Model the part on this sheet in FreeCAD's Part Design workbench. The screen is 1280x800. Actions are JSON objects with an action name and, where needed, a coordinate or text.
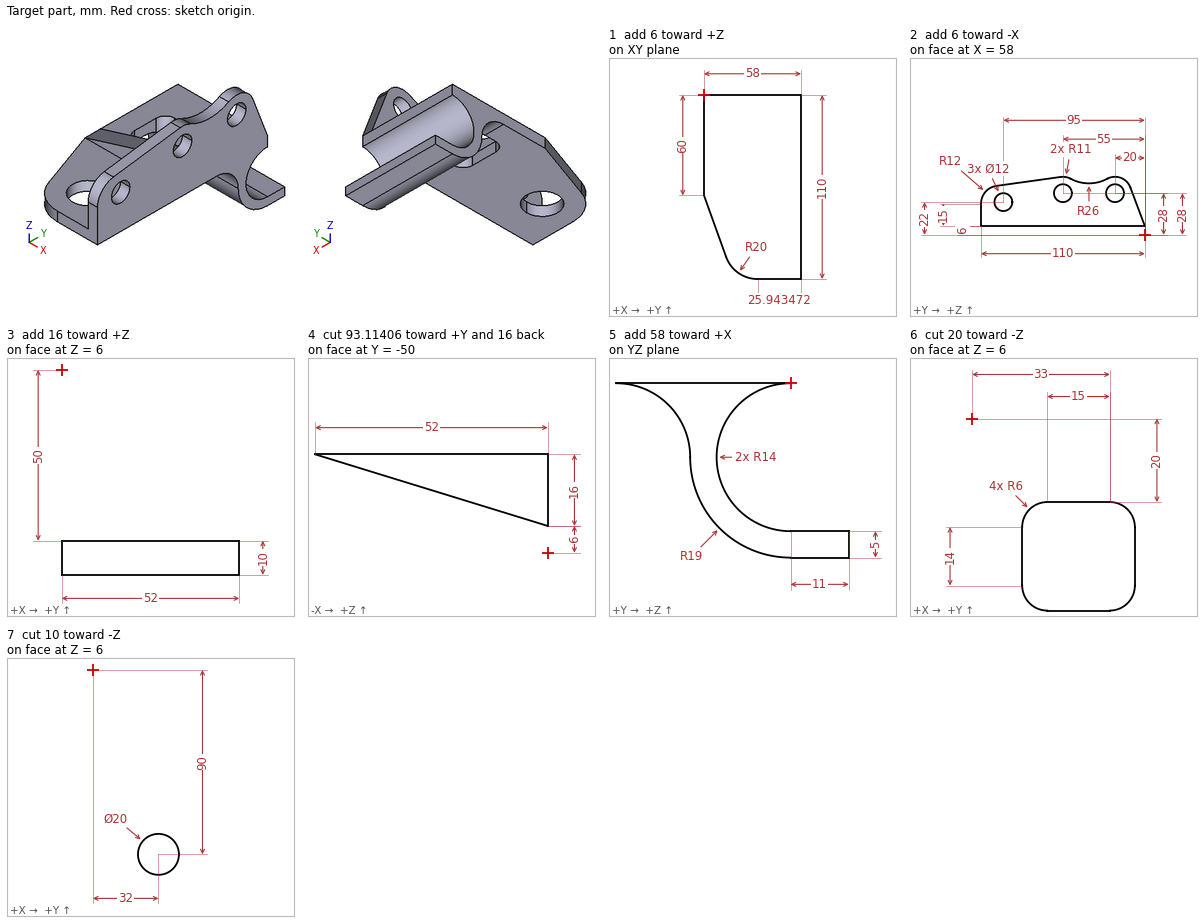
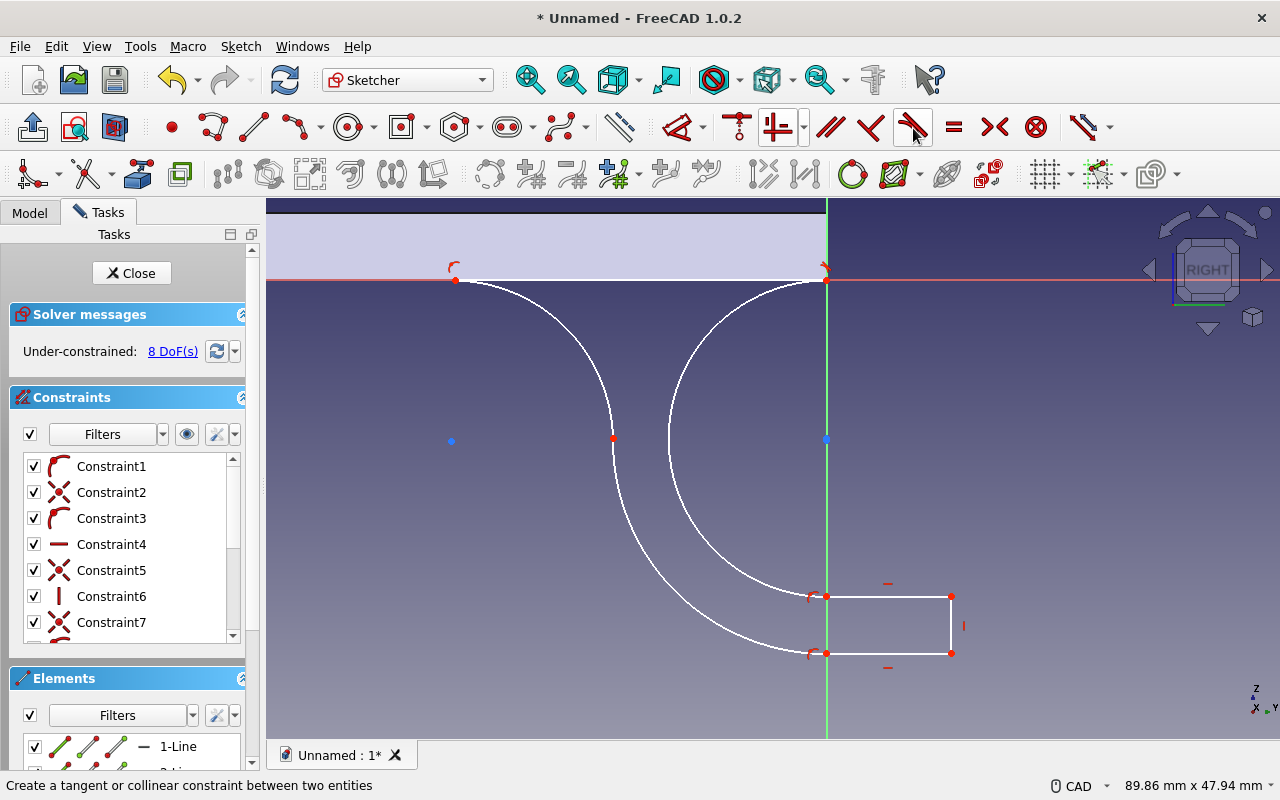
{"action": "left_click", "coordinate": [567, 280]}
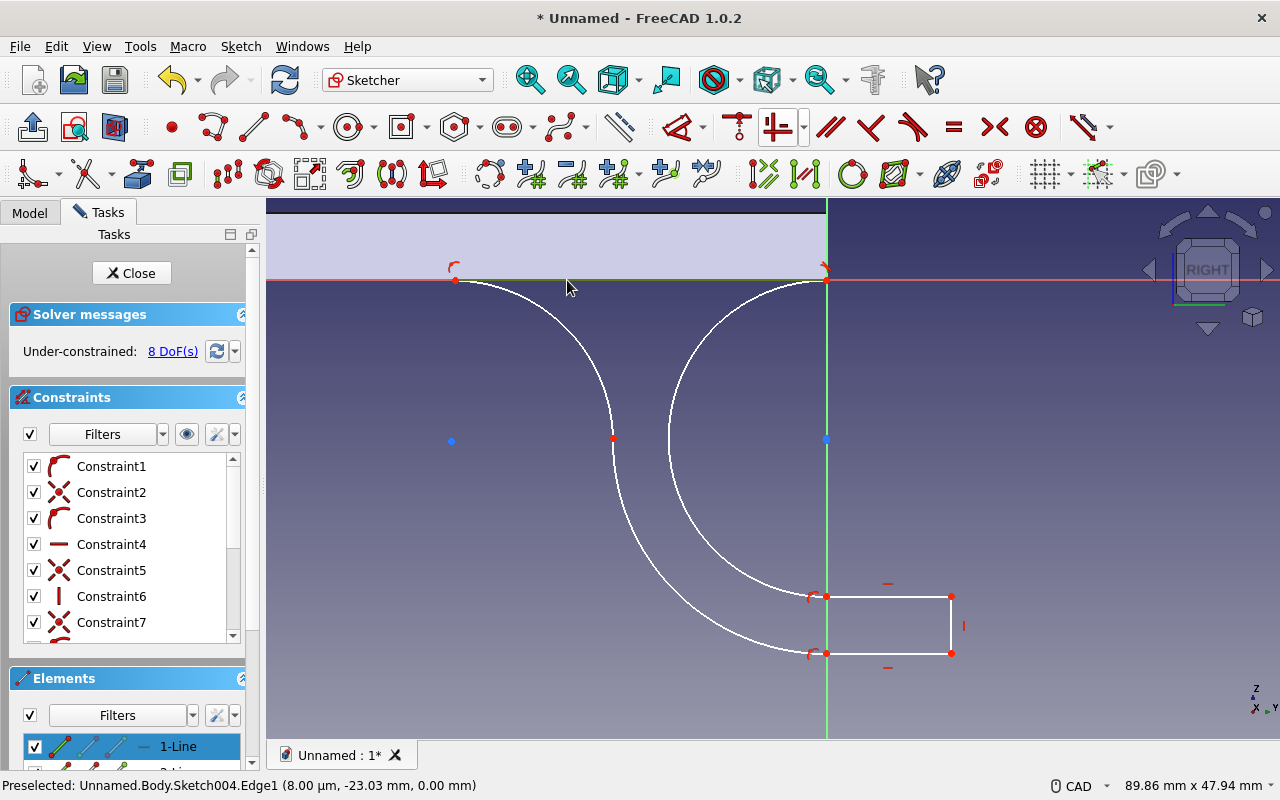
{"action": "left_click", "coordinate": [595, 368]}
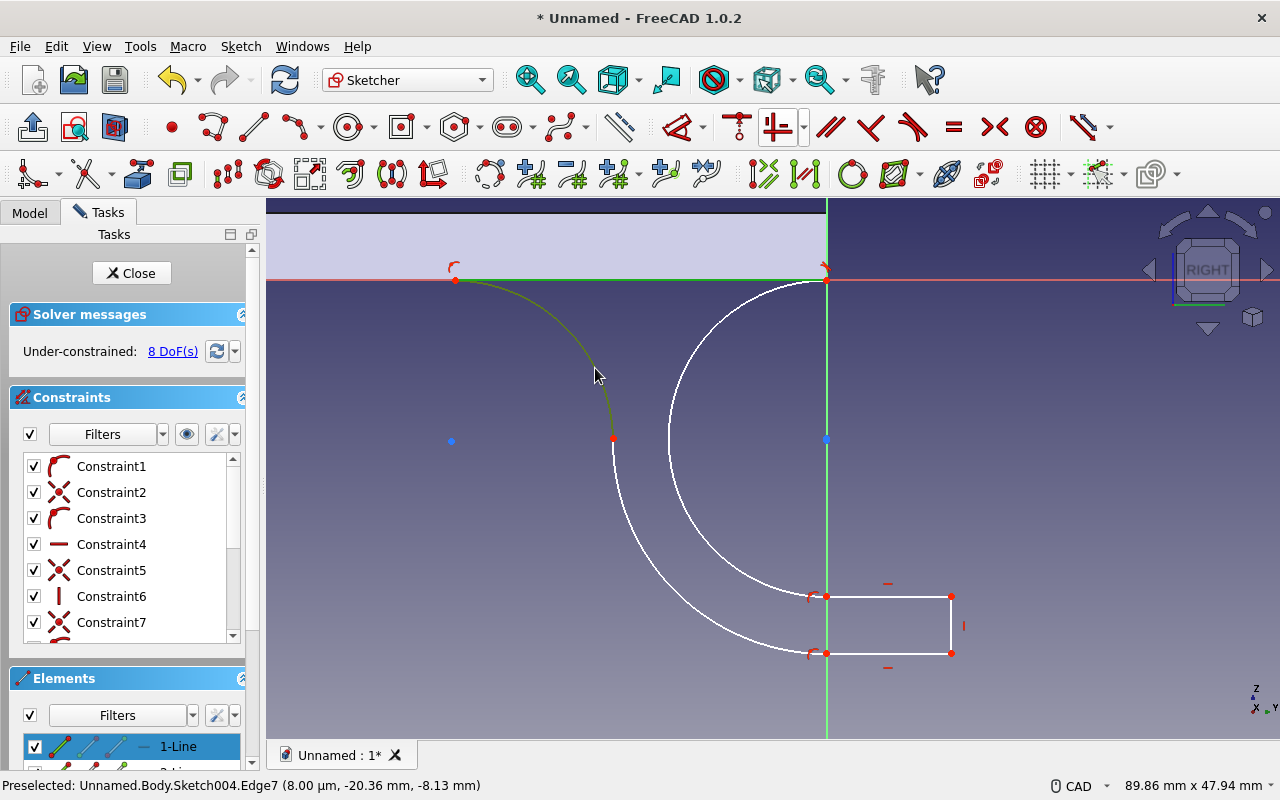
{"action": "left_click", "coordinate": [913, 128]}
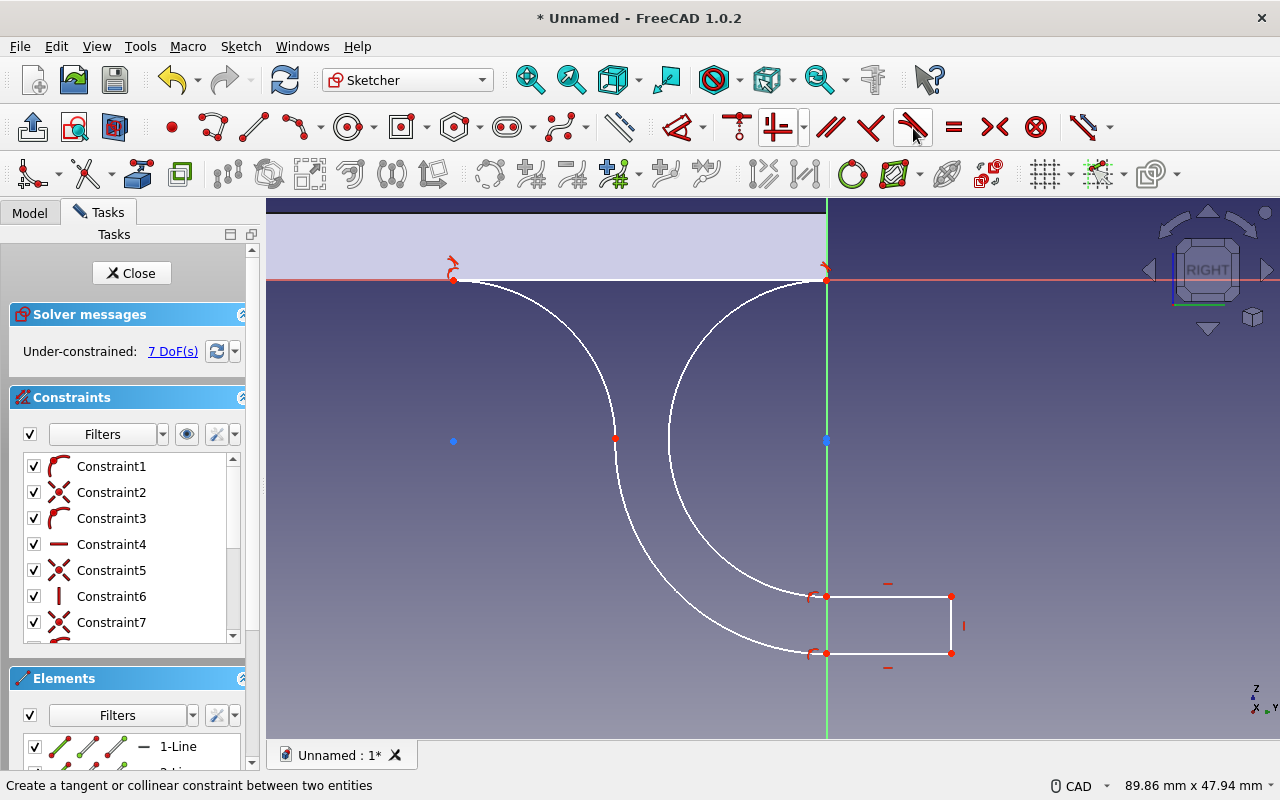
{"action": "left_click", "coordinate": [914, 654]}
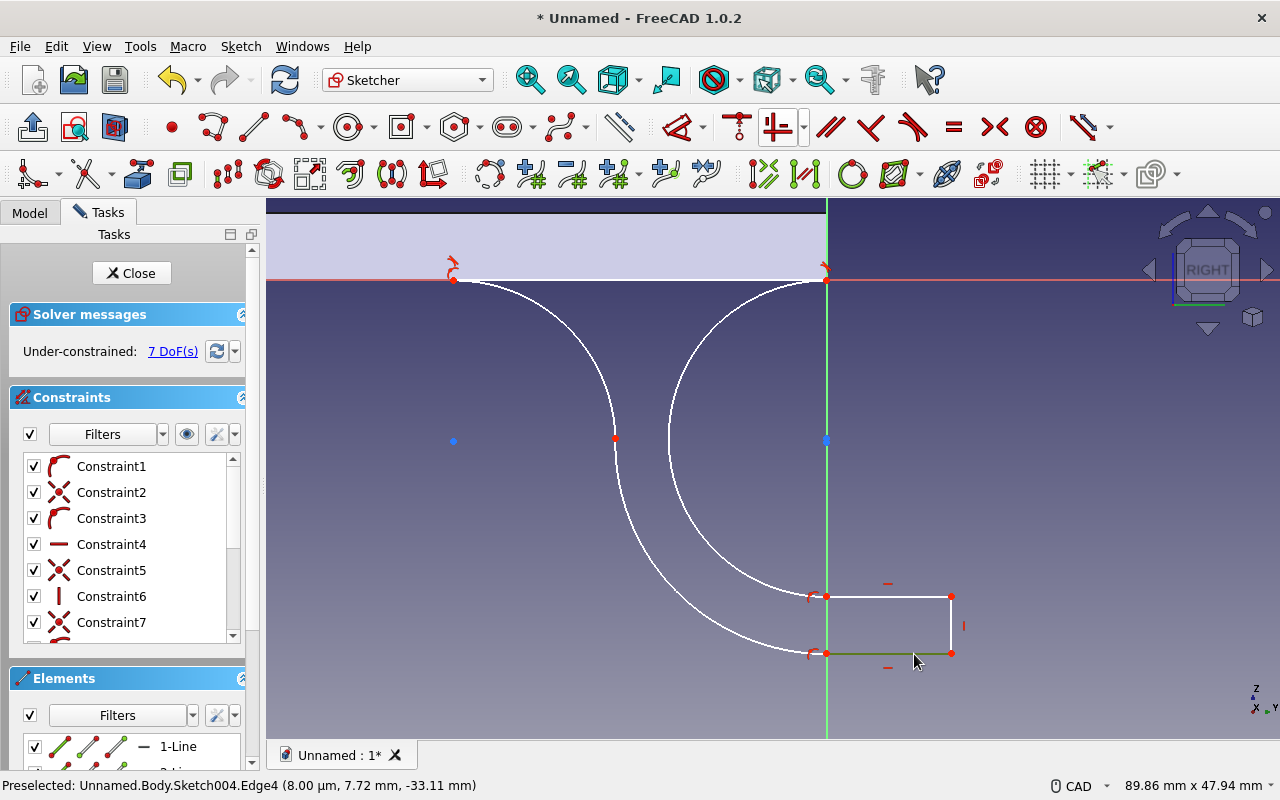
{"action": "left_click", "coordinate": [637, 536]}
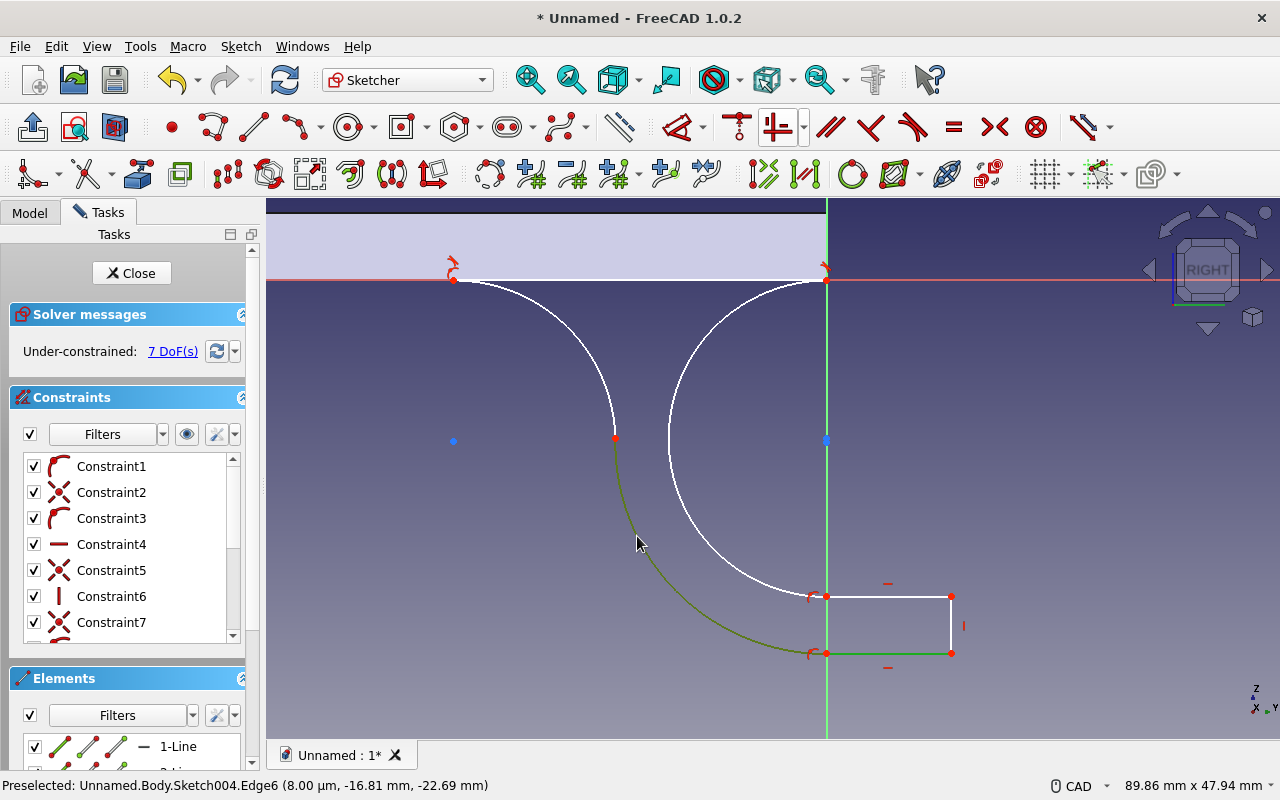
{"action": "left_click", "coordinate": [913, 128]}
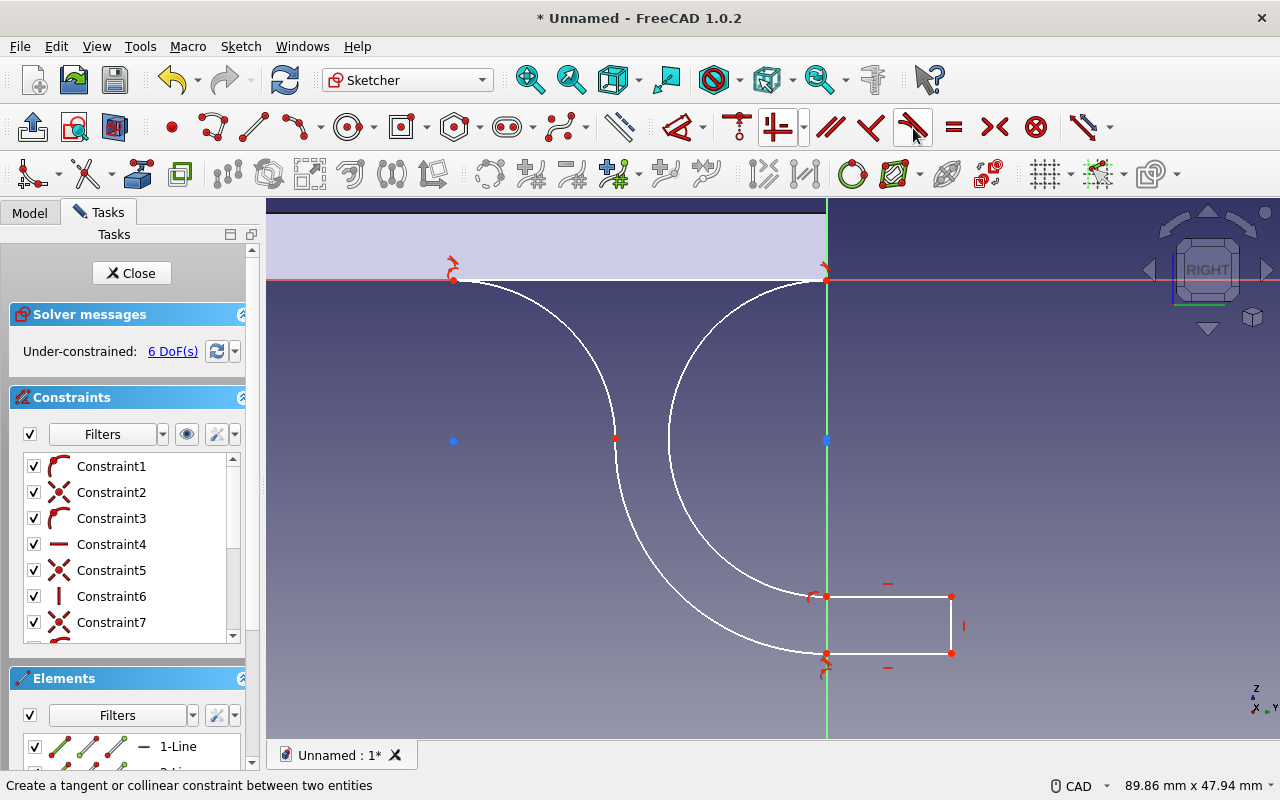
{"action": "left_click", "coordinate": [637, 536]}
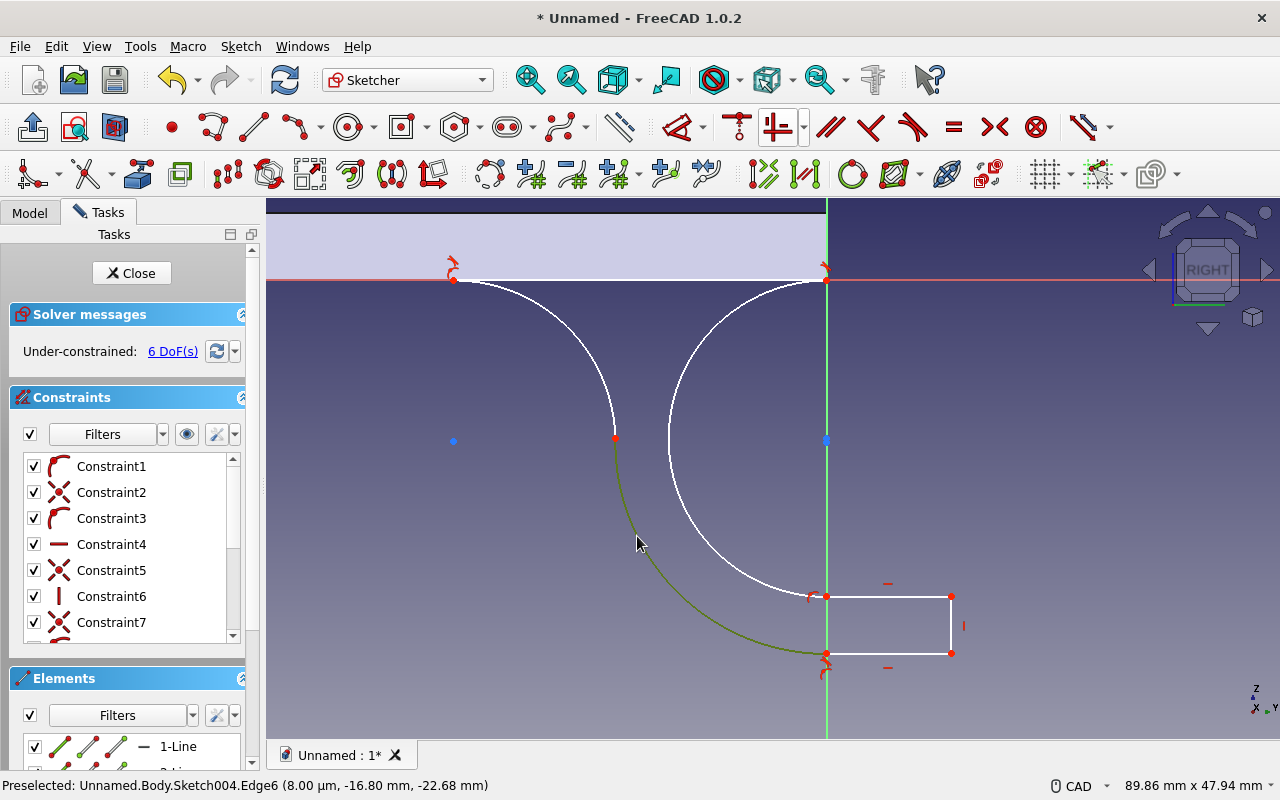
{"action": "left_click", "coordinate": [597, 367]}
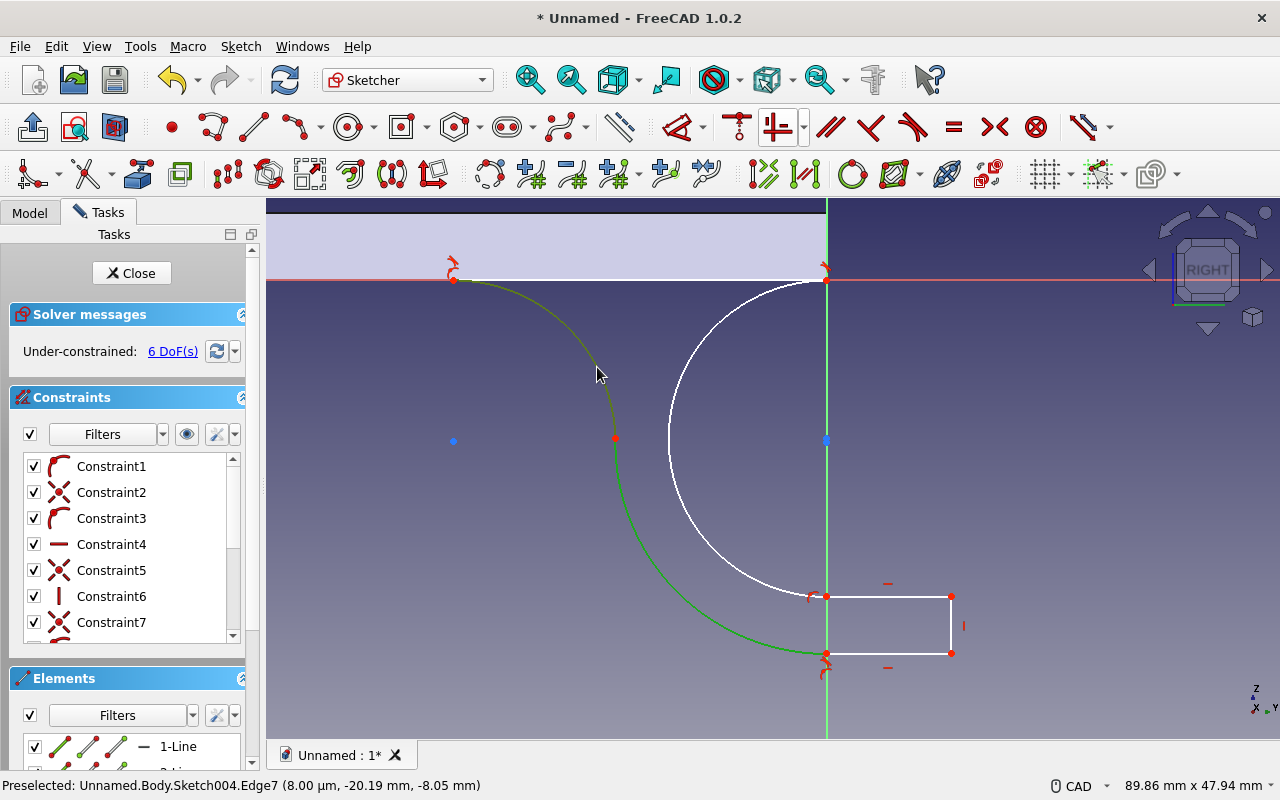
{"action": "left_click", "coordinate": [913, 128]}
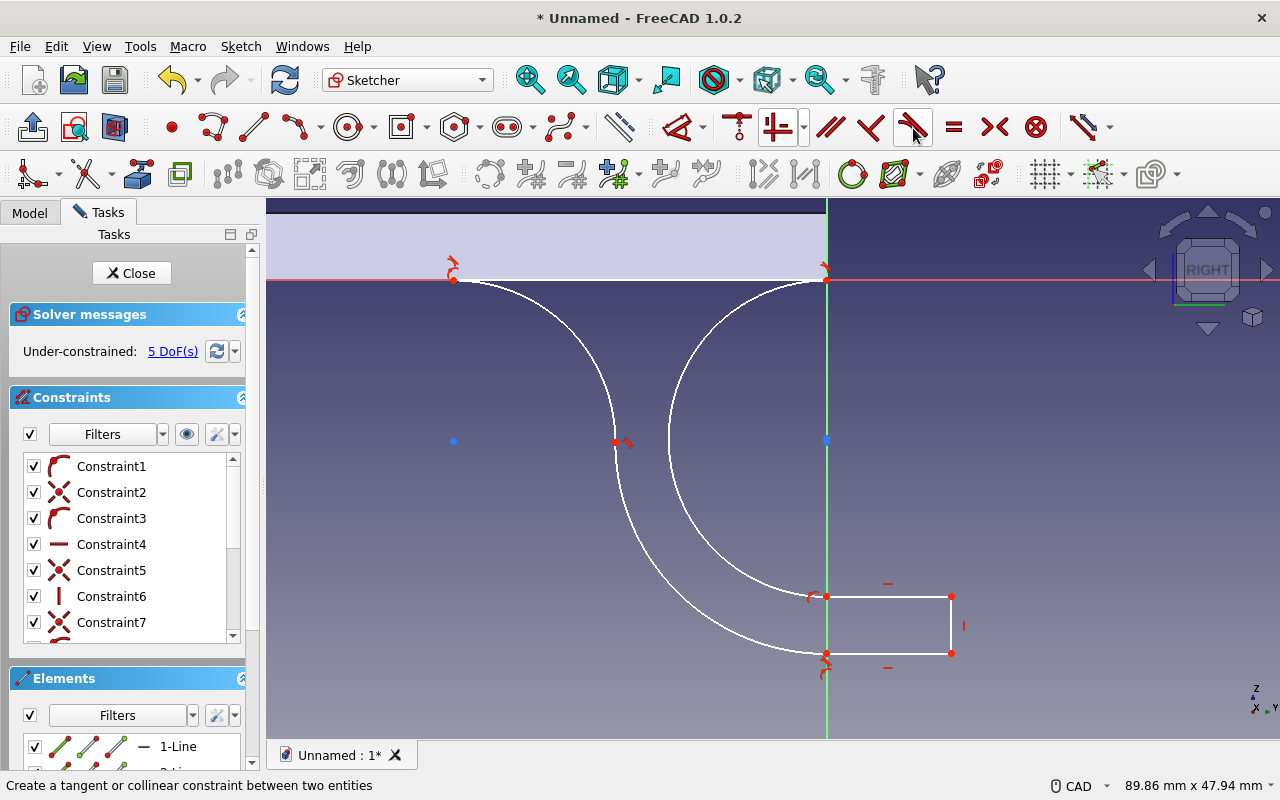
{"action": "left_click", "coordinate": [699, 346]}